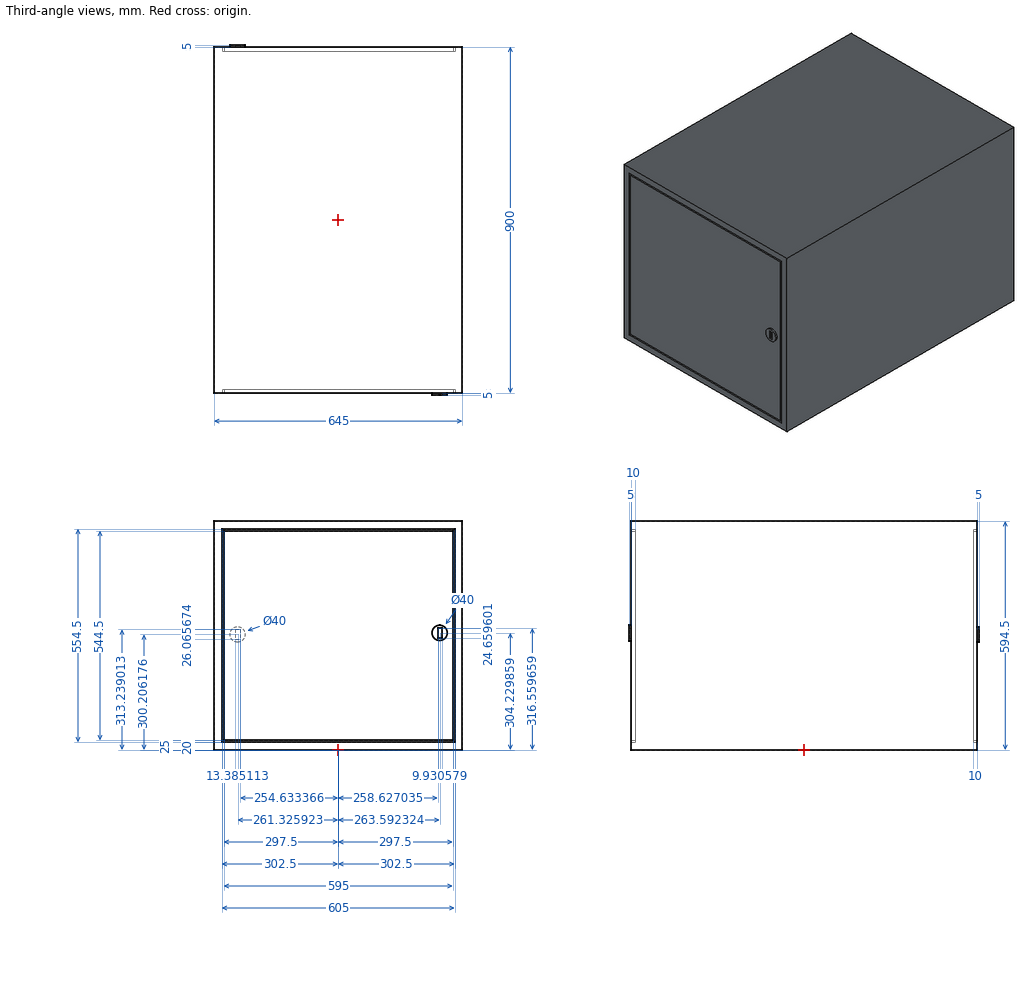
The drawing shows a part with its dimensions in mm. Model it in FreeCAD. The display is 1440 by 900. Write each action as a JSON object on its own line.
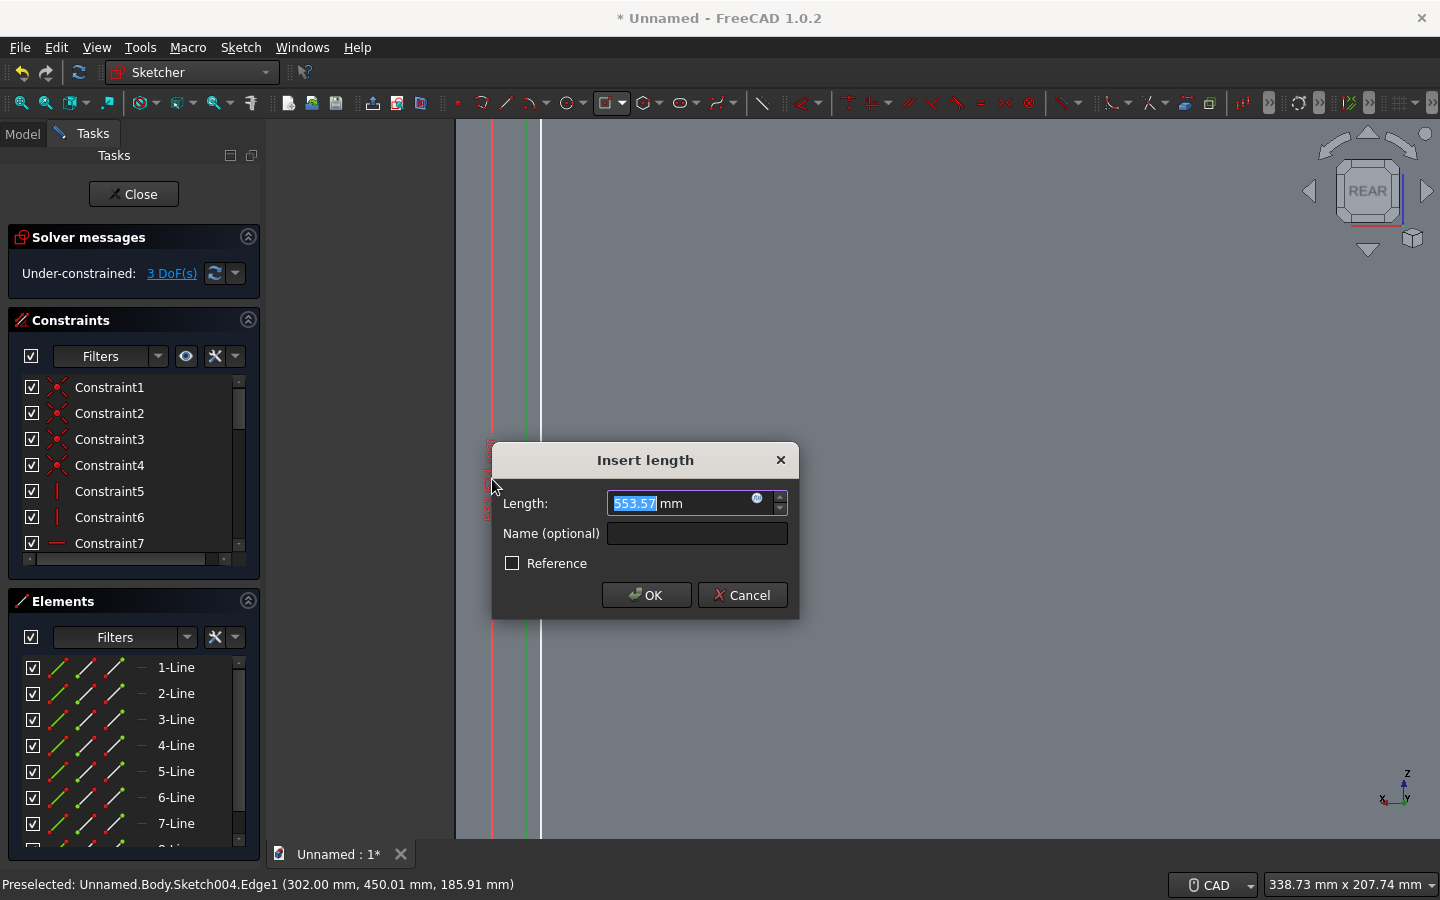
{"action": "type", "text": "554.5"}
{"action": "key", "text": "Return"}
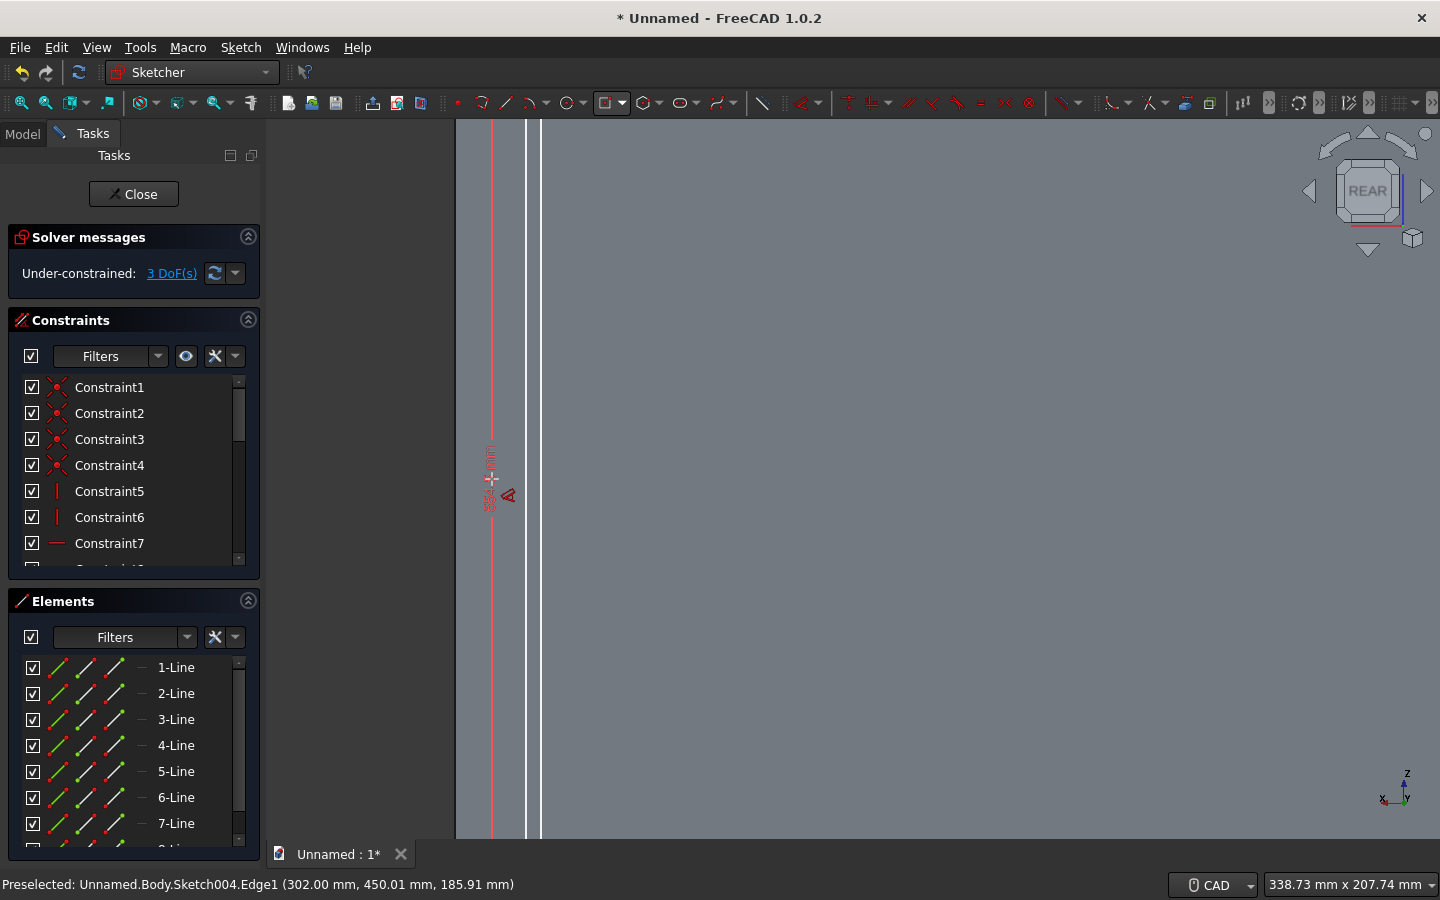
{"action": "left_click", "coordinate": [541, 311]}
{"action": "left_click", "coordinate": [507, 326]}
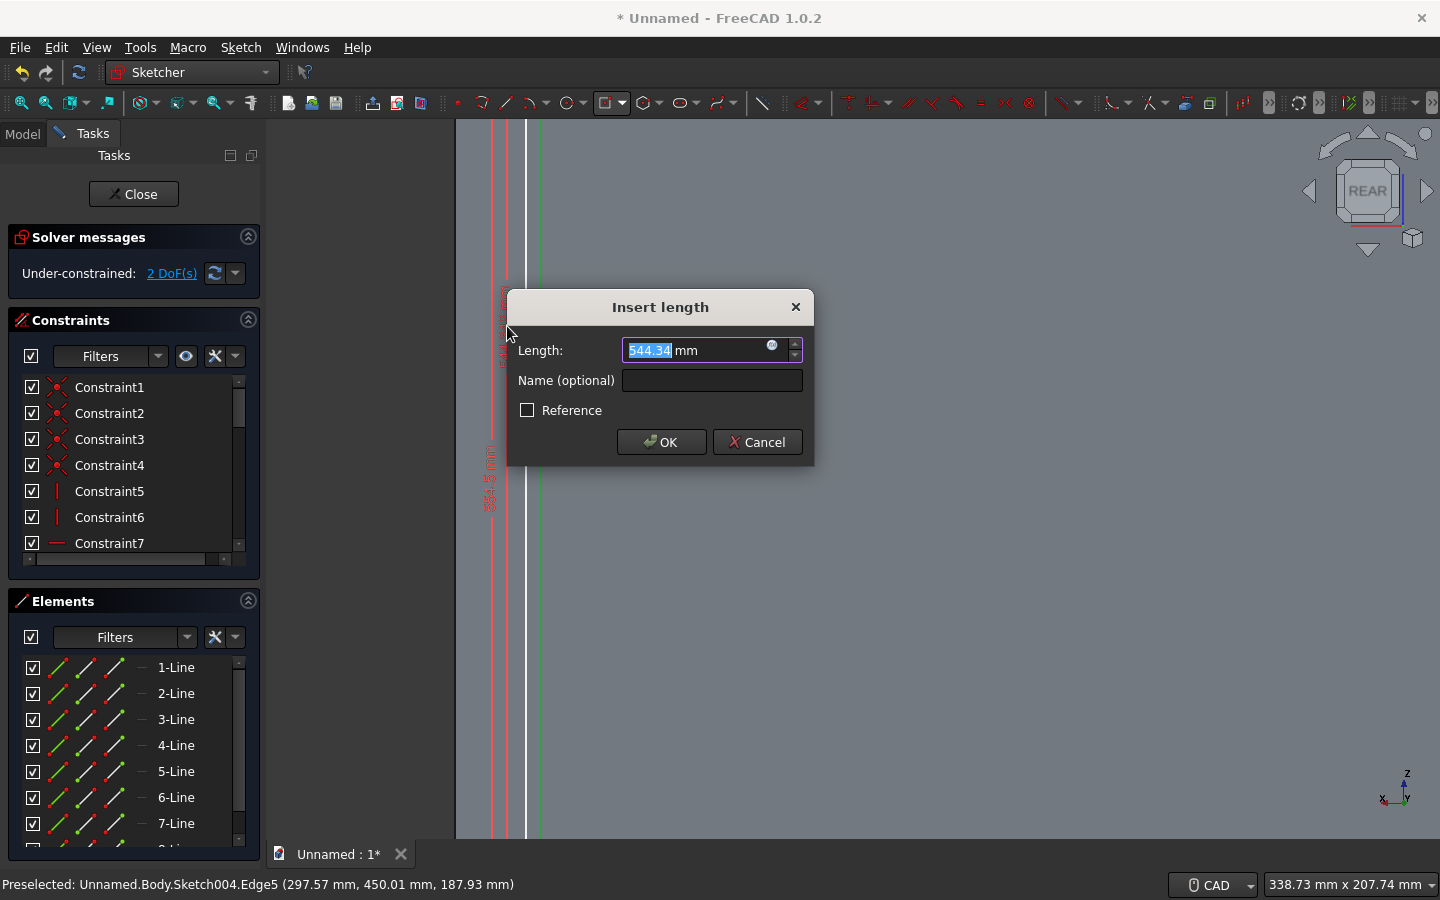
{"action": "type", "text": "544.5"}
{"action": "key", "text": "Return"}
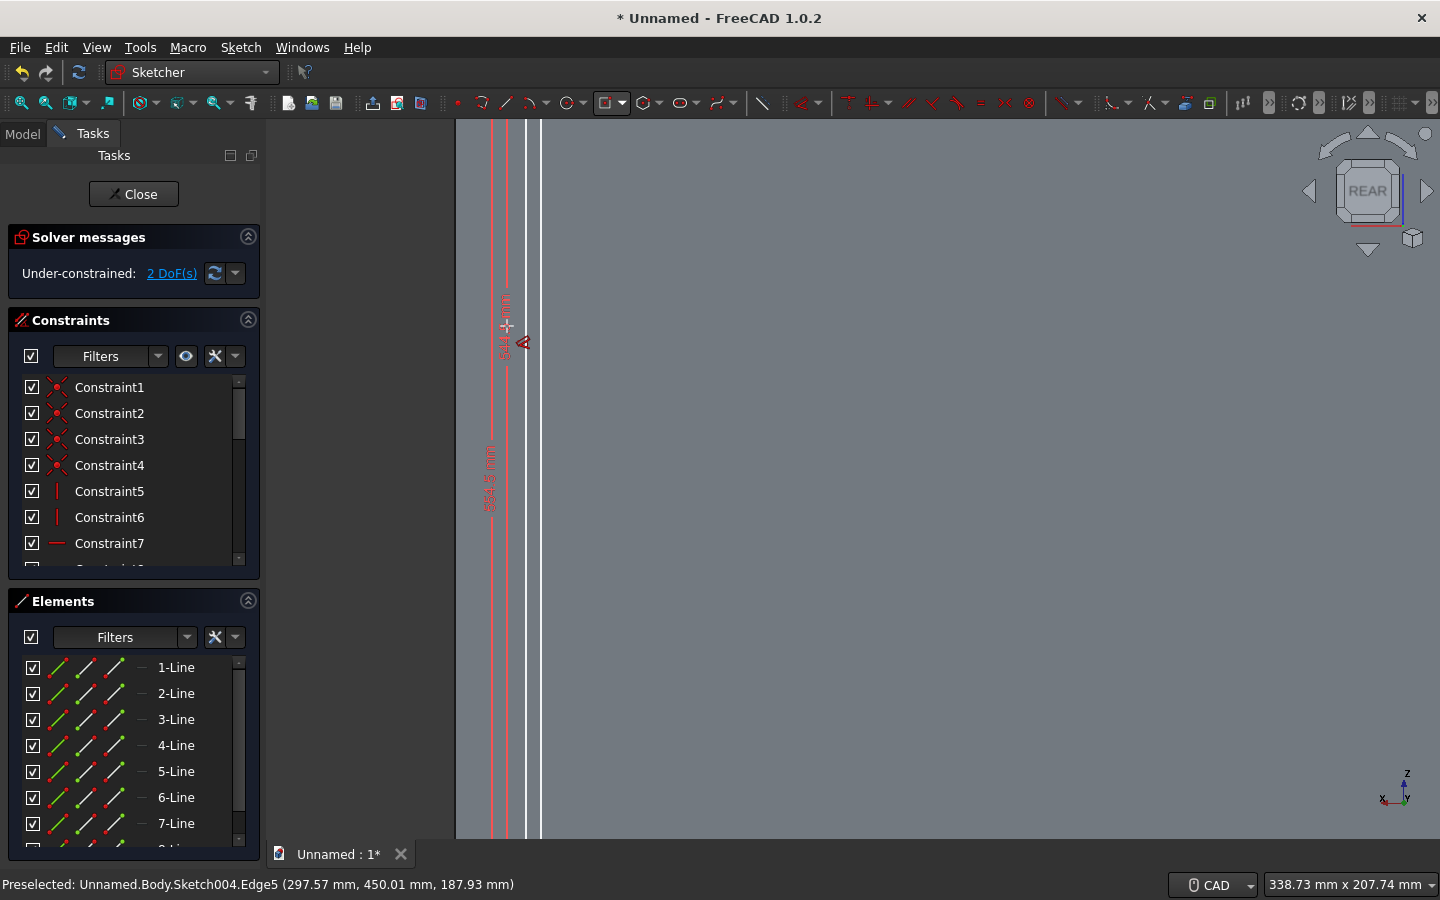
{"action": "scroll", "coordinate": [527, 646], "scroll_direction": "down", "scroll_amount": 7}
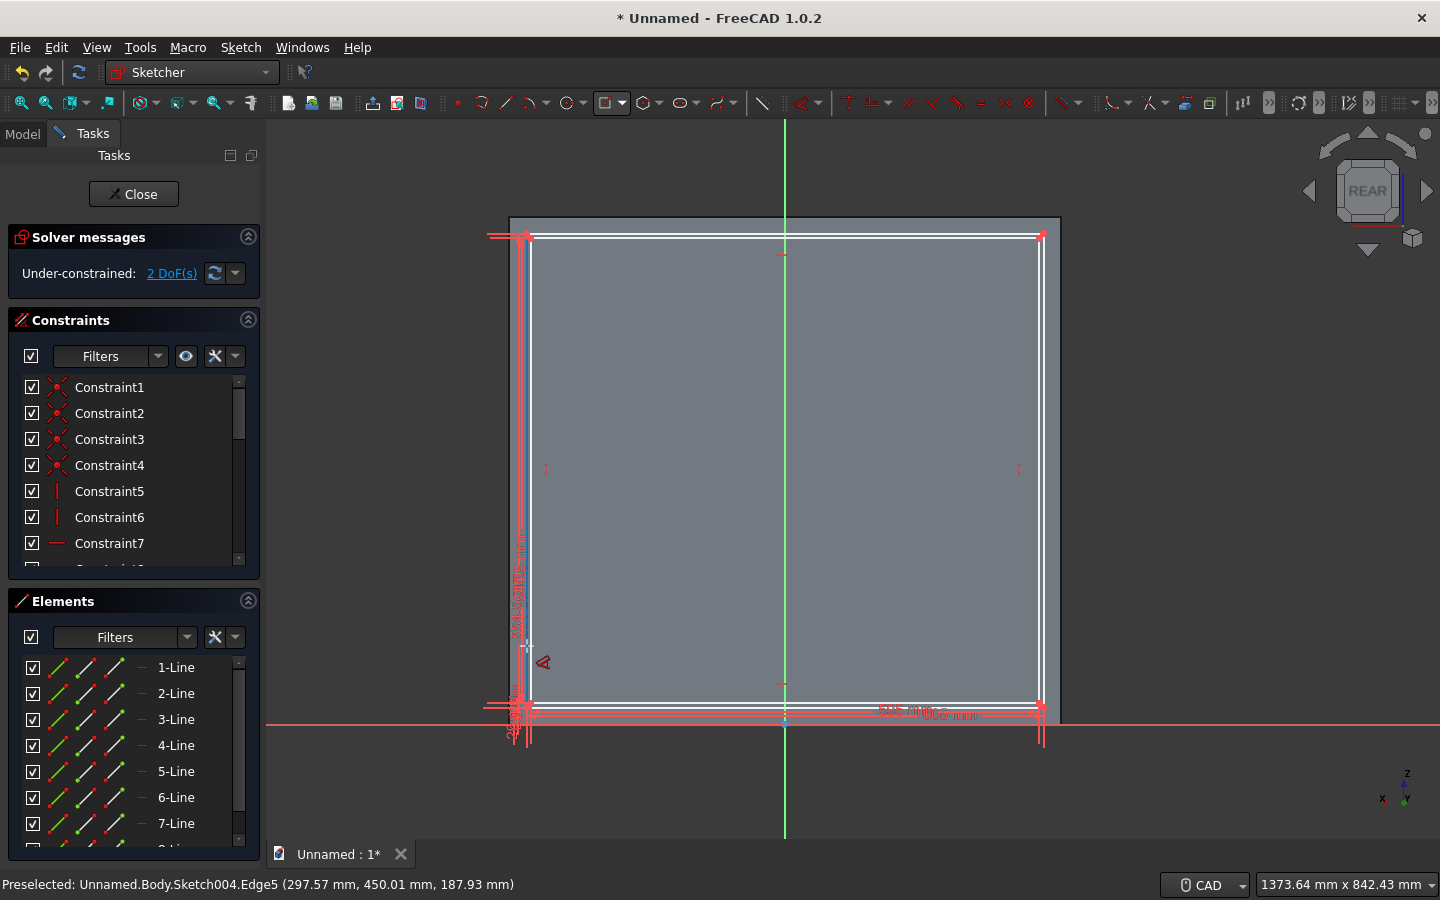
{"action": "scroll", "coordinate": [527, 234], "scroll_direction": "up", "scroll_amount": 4}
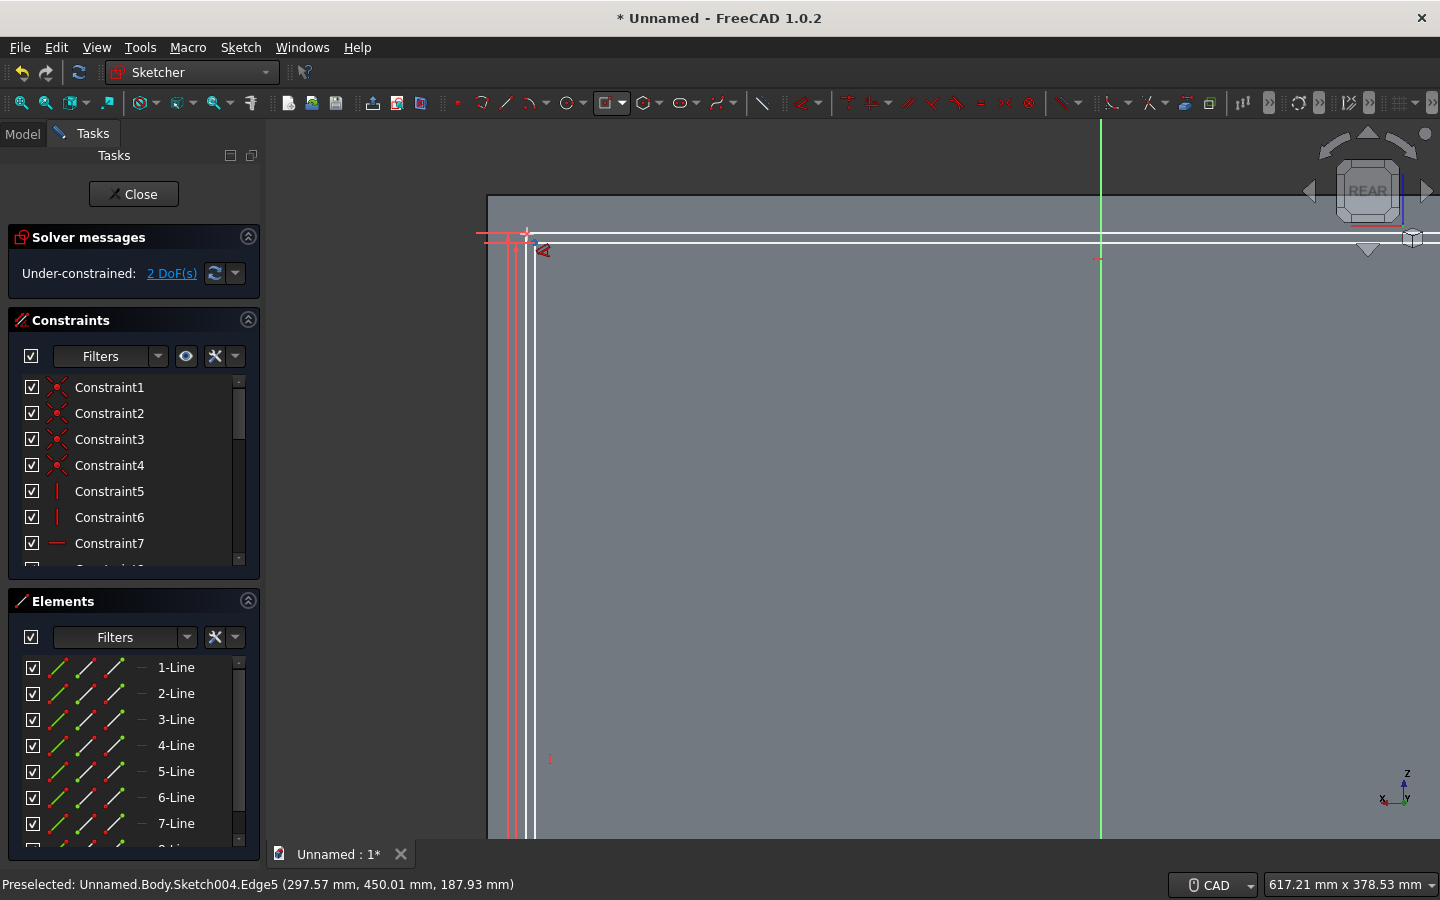
{"action": "left_click", "coordinate": [526, 233]}
{"action": "left_click", "coordinate": [814, 199]}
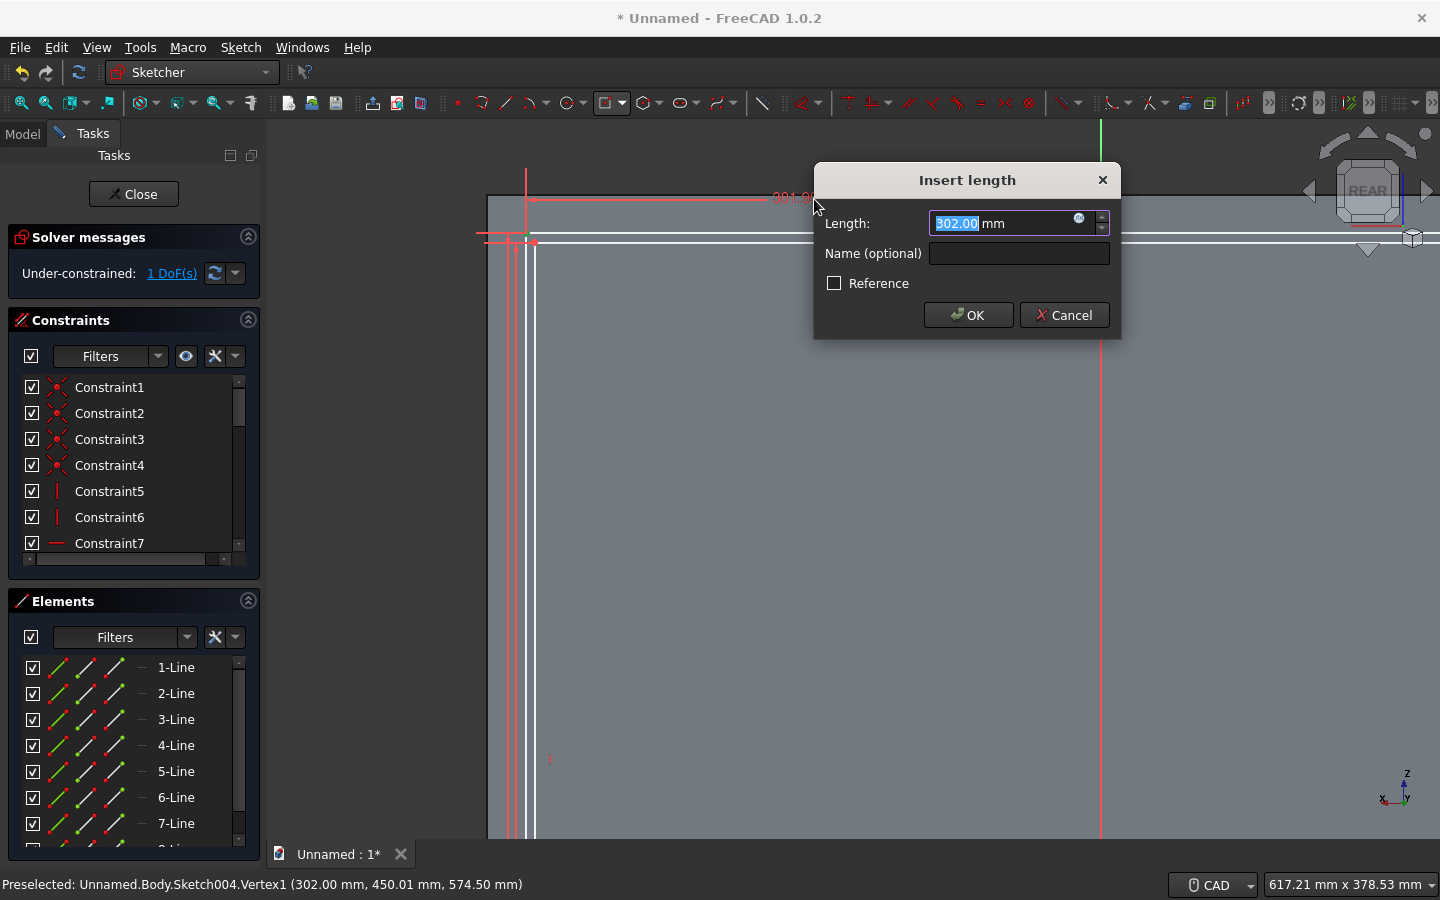
{"action": "type", "text": "302.5"}
{"action": "key", "text": "Return"}